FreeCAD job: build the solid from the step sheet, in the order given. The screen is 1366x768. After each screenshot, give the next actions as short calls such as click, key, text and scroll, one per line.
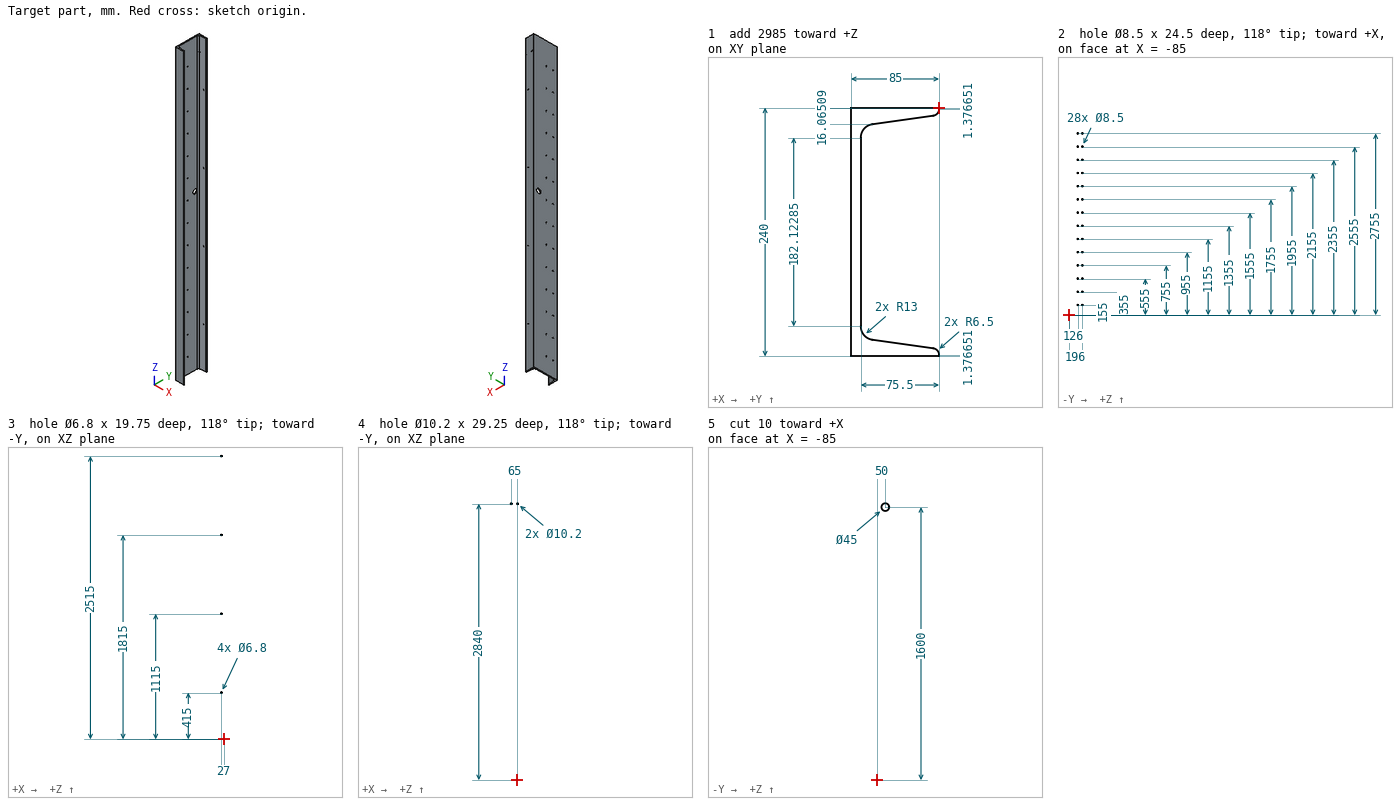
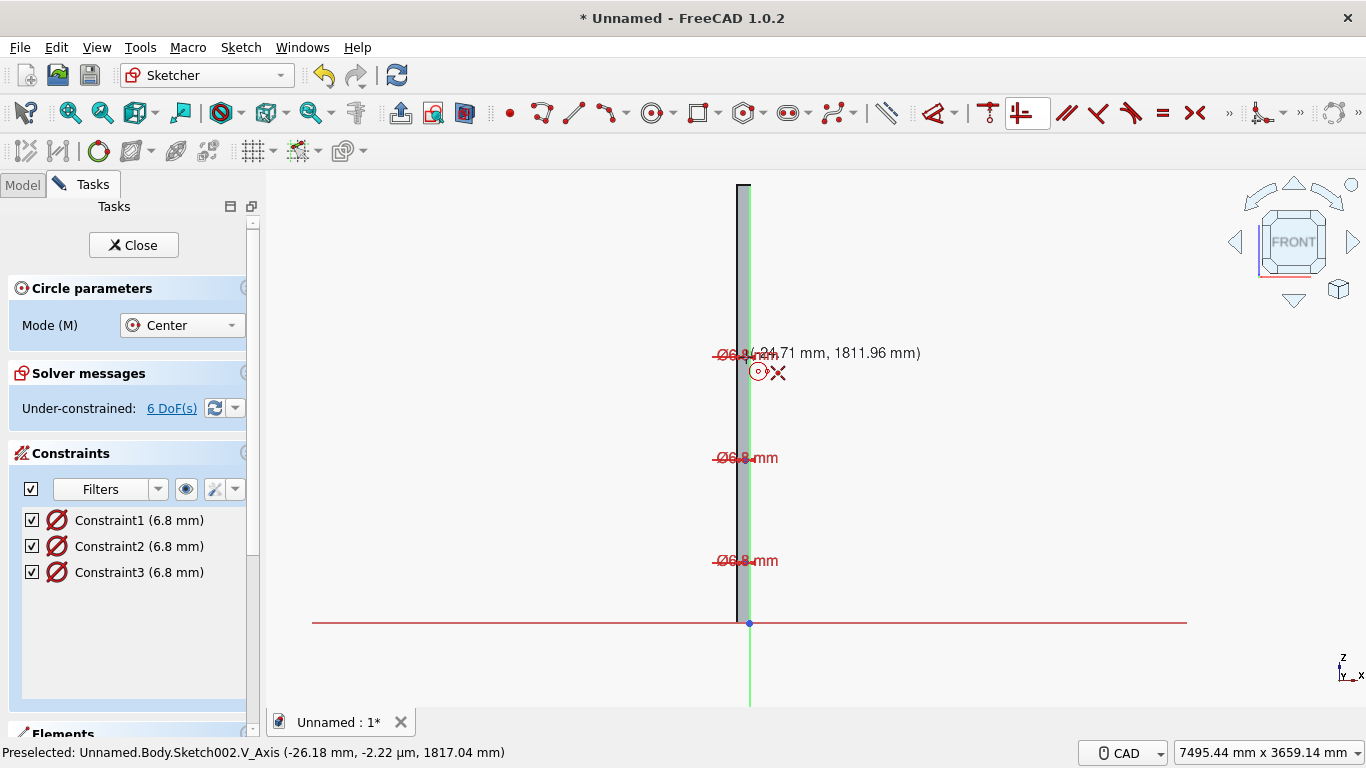
scroll(746, 254, up, 20)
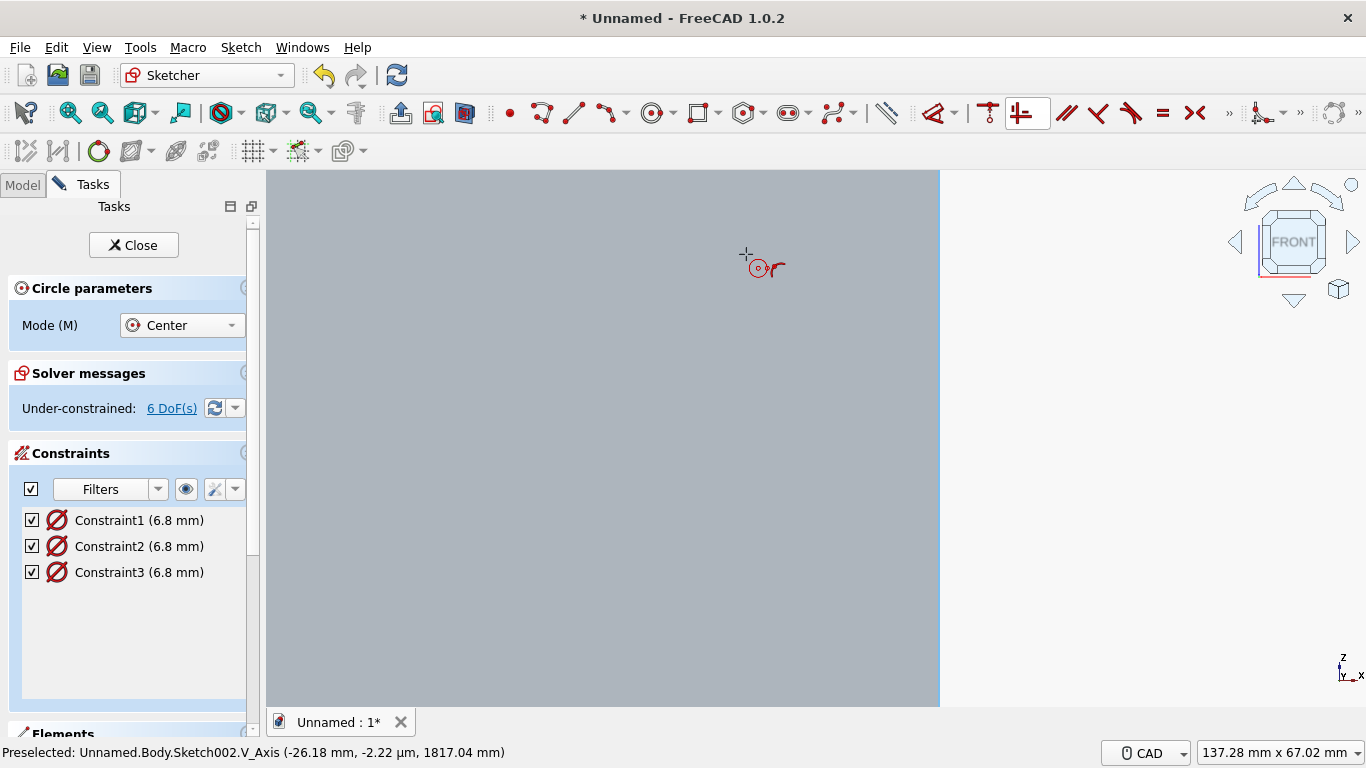
scroll(748, 438, down, 15)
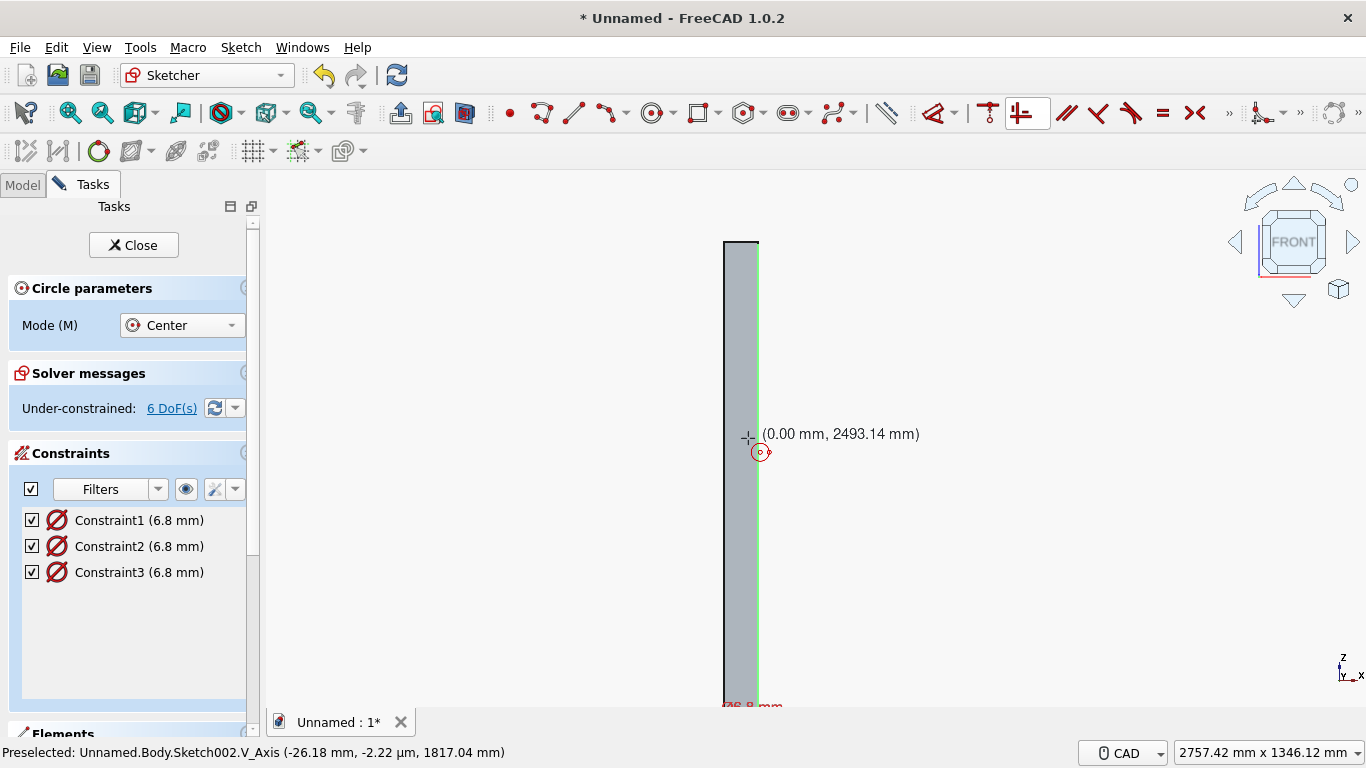
scroll(745, 198, down, 5)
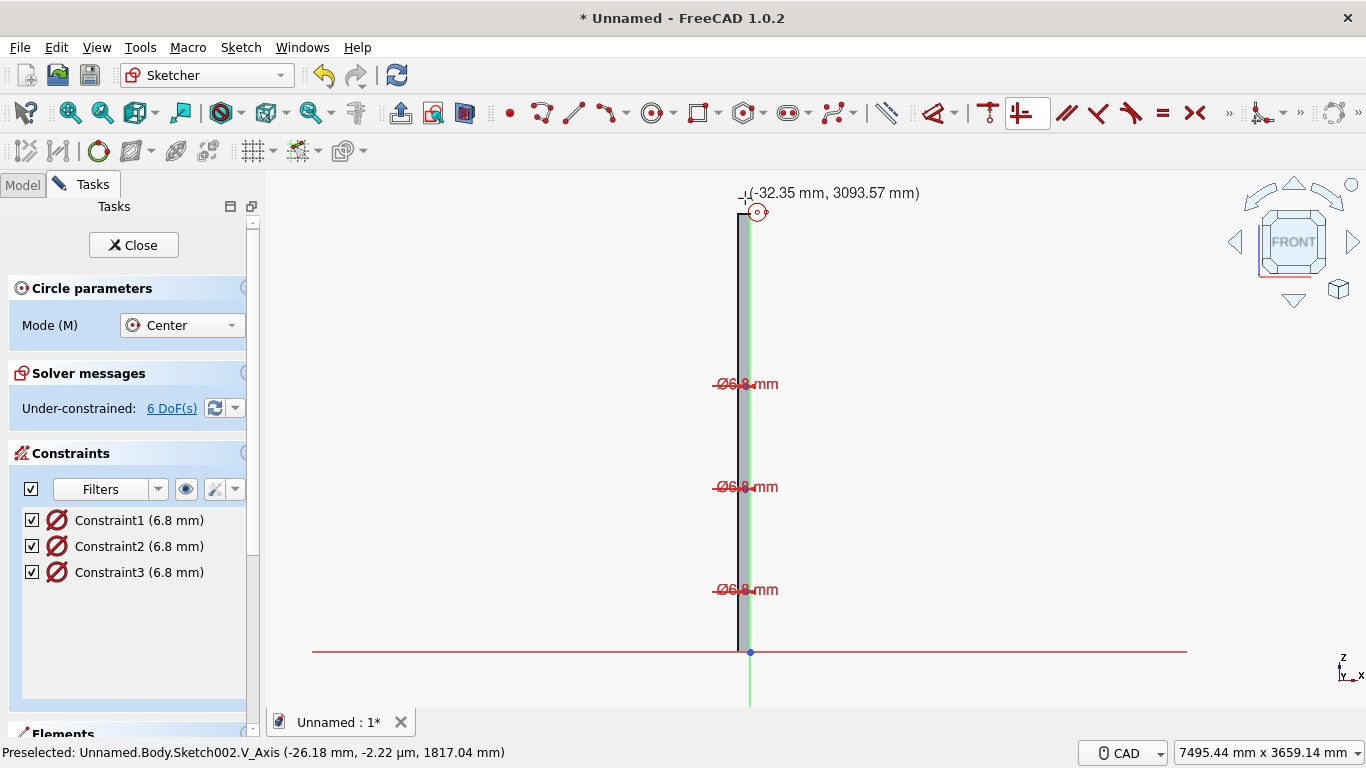
scroll(746, 283, up, 7)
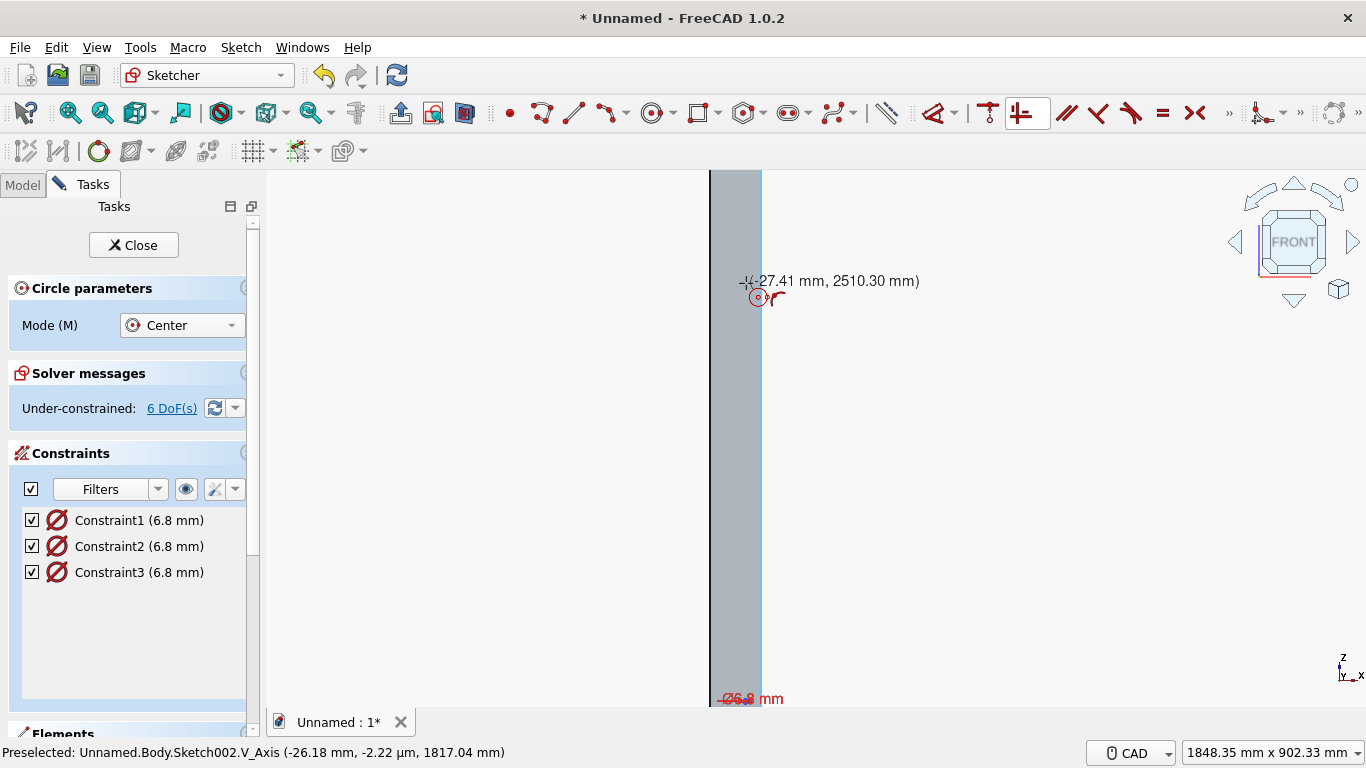
click(745, 284)
move(746, 282)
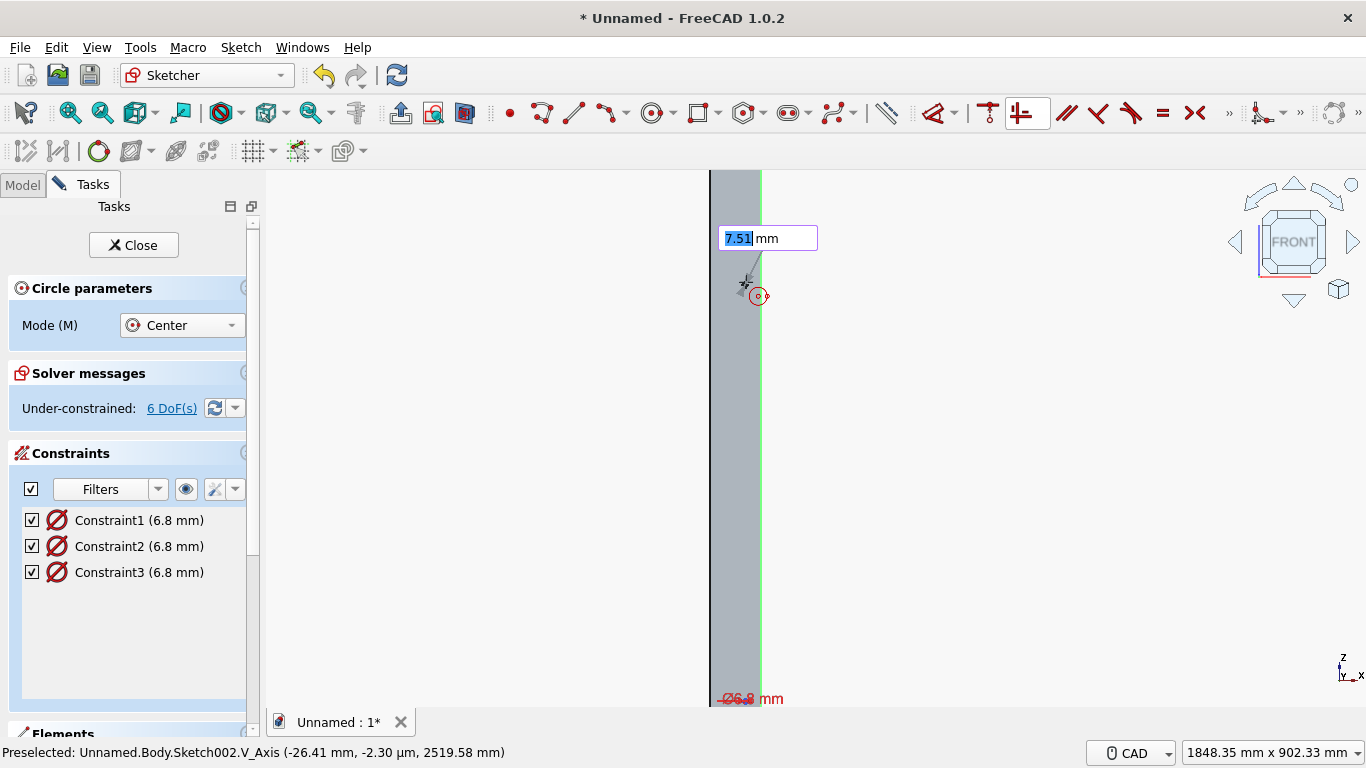
text(6.8)
key(Return)
key(Escape)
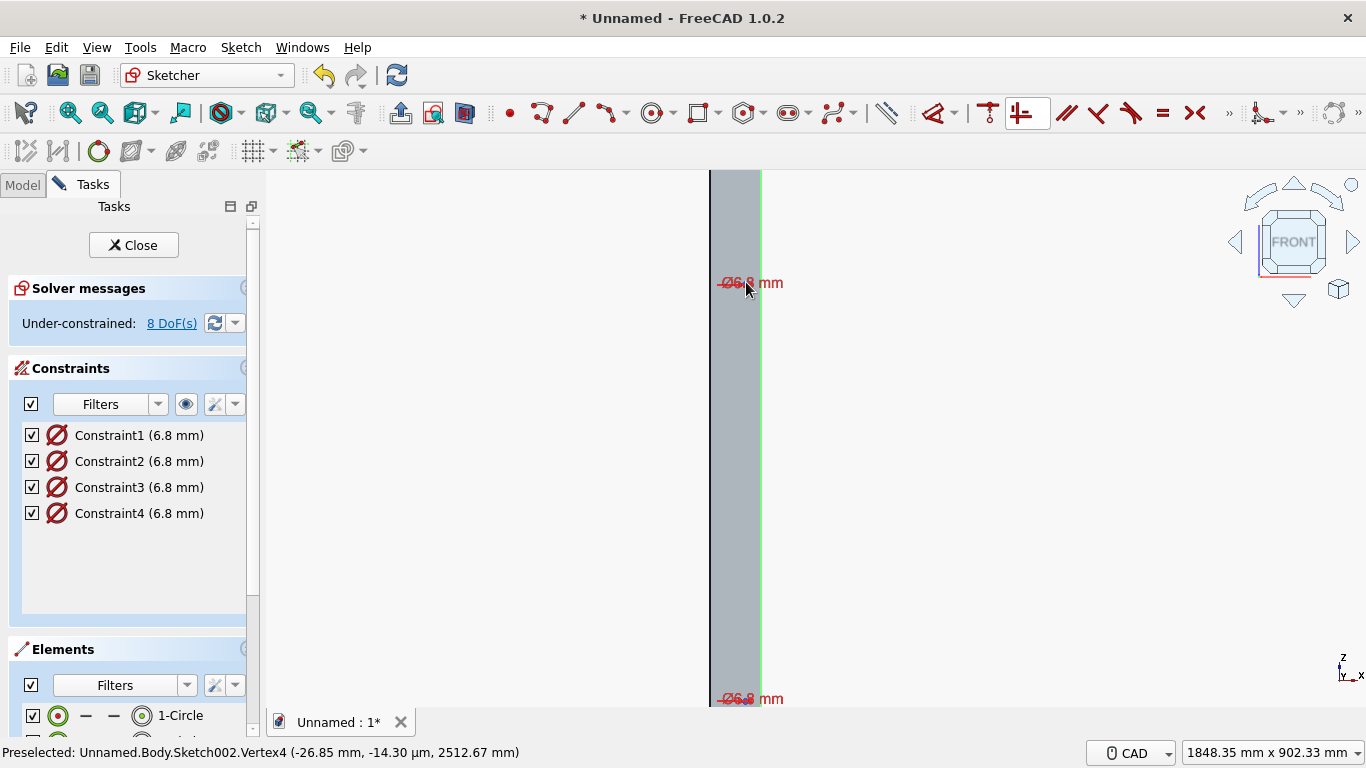
scroll(746, 245, down, 7)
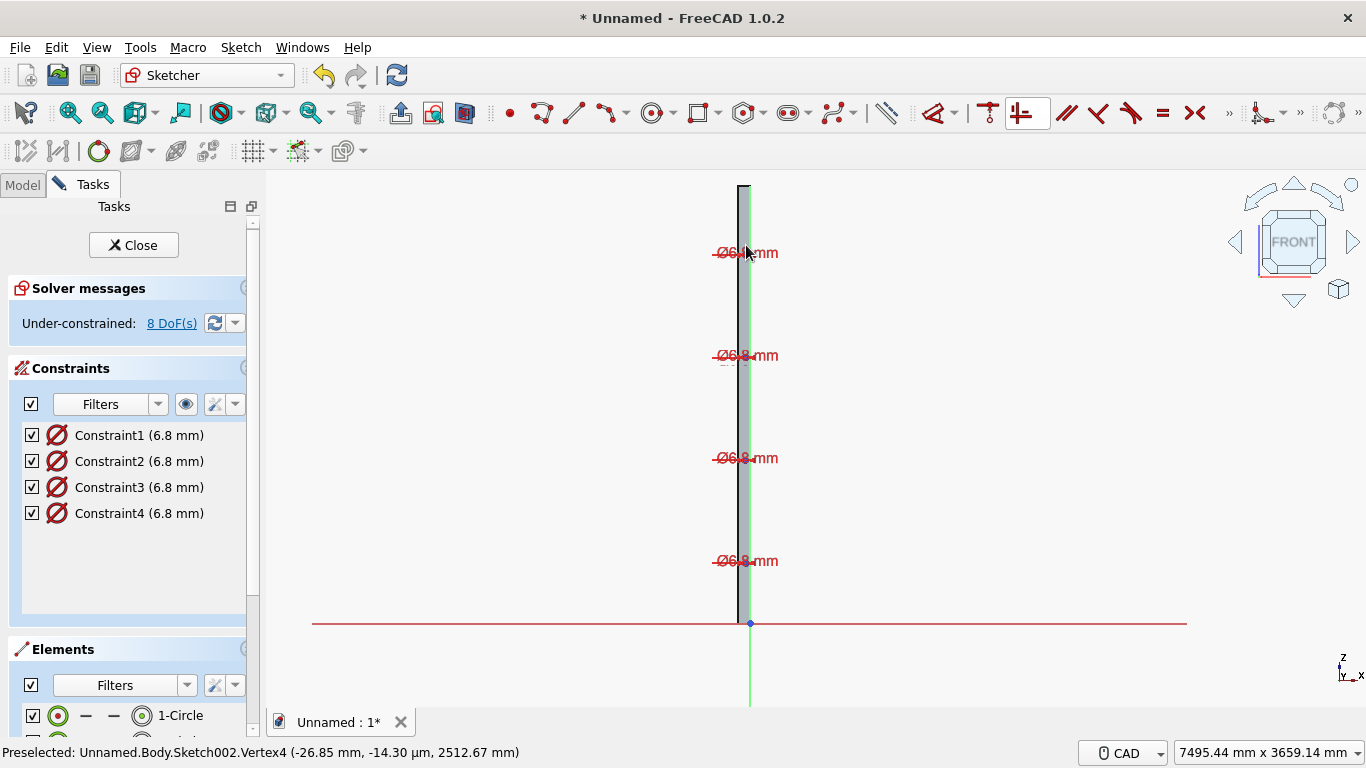
click(746, 563)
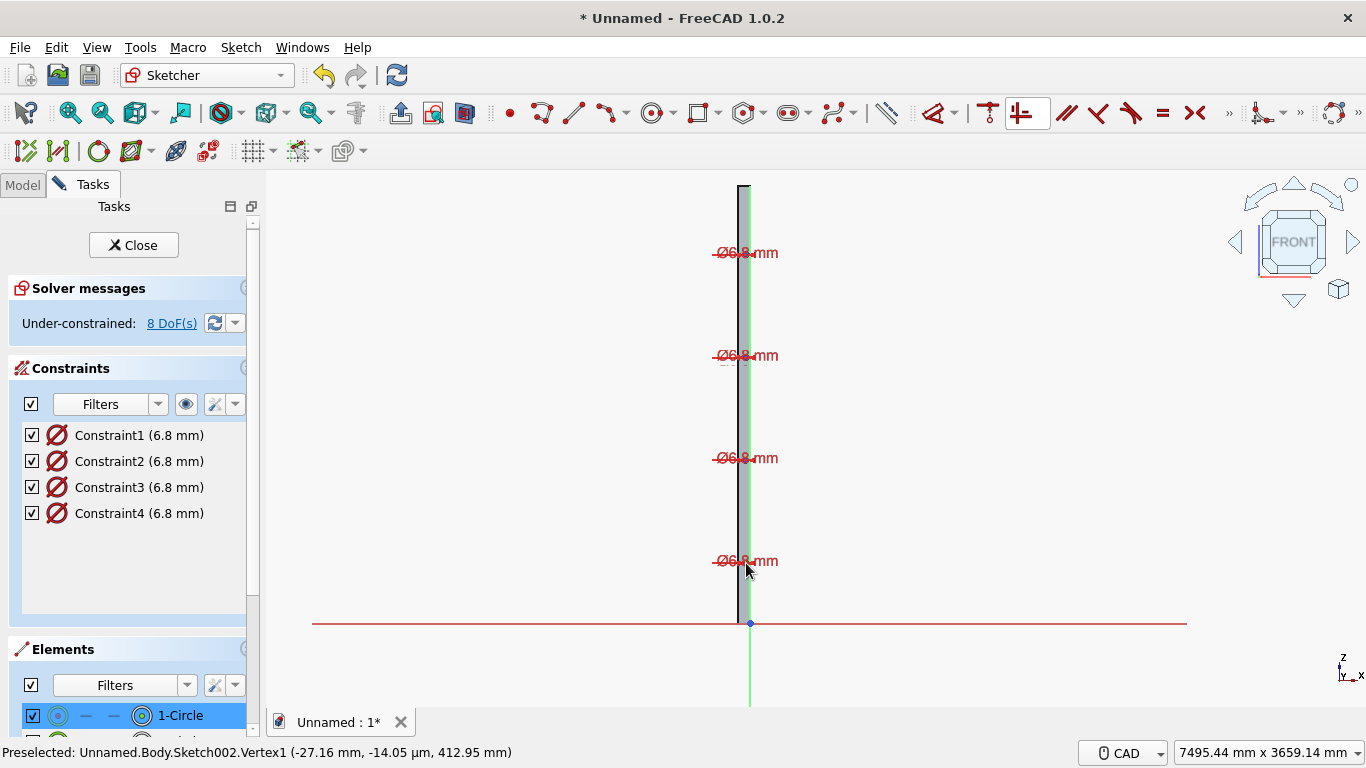
click(746, 460)